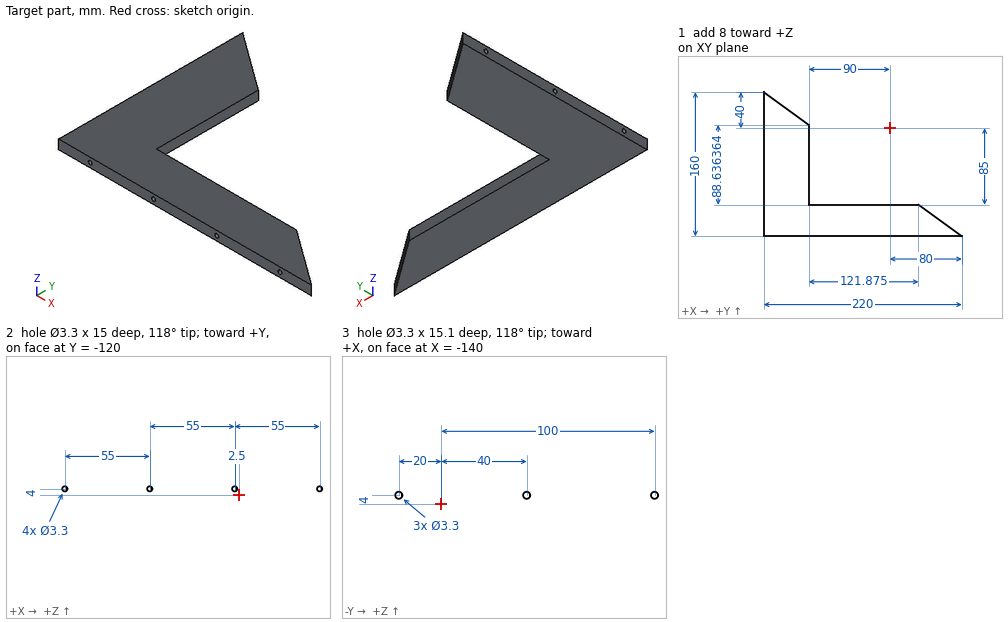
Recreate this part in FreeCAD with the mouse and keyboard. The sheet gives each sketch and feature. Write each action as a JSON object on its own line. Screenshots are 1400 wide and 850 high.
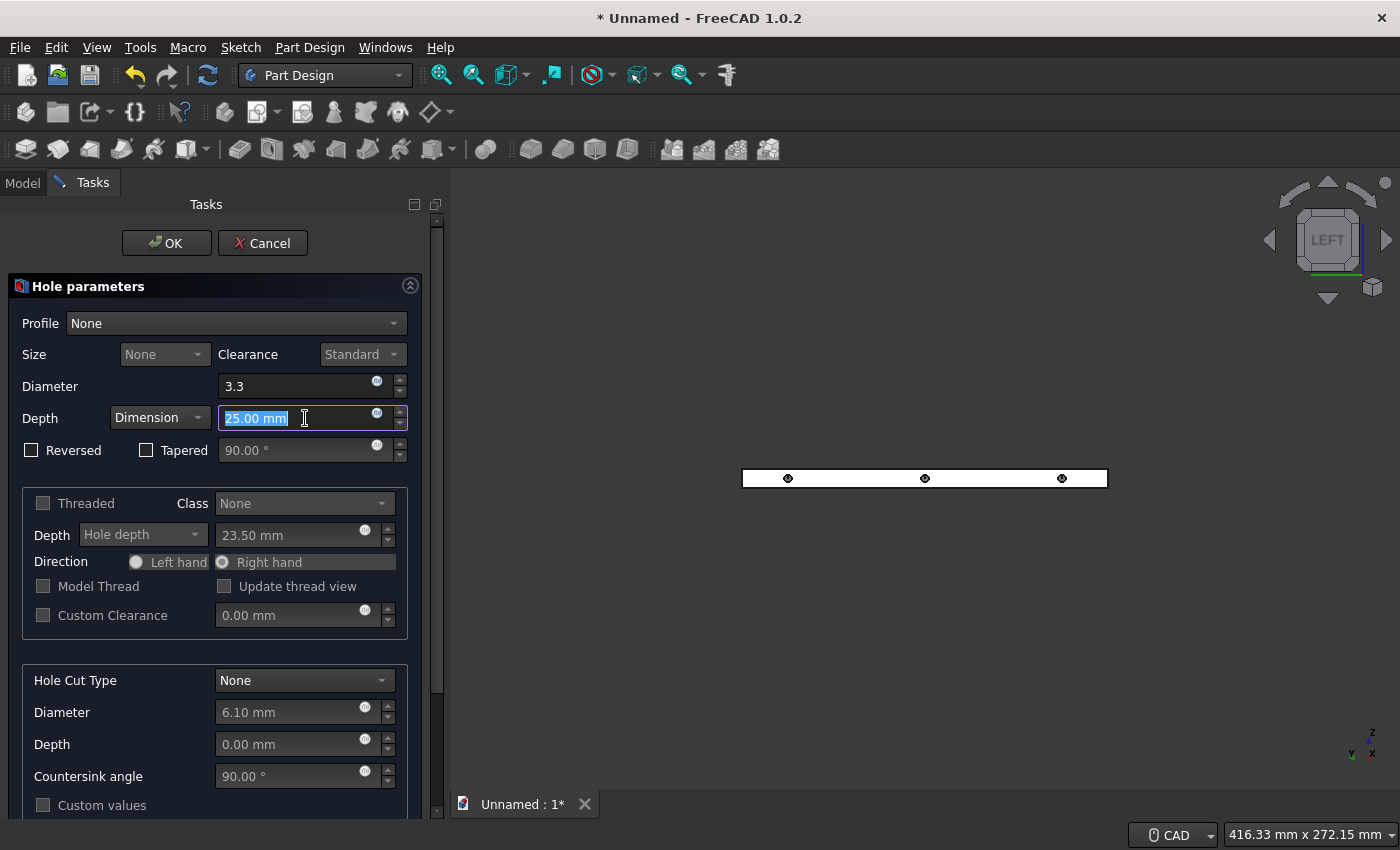
{"action": "type", "text": "15.1"}
{"action": "key", "text": "Tab"}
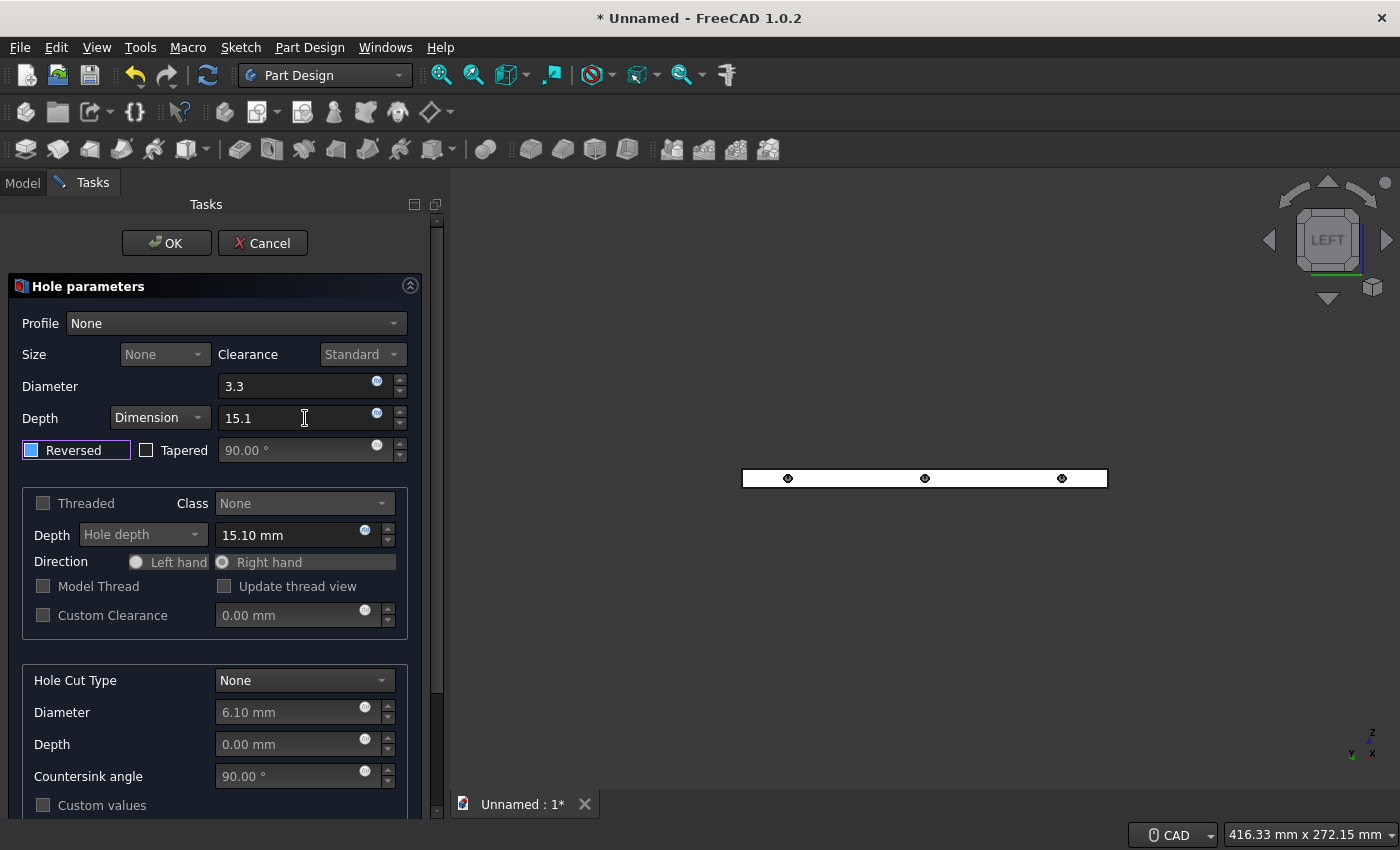
{"action": "left_click", "coordinate": [167, 243]}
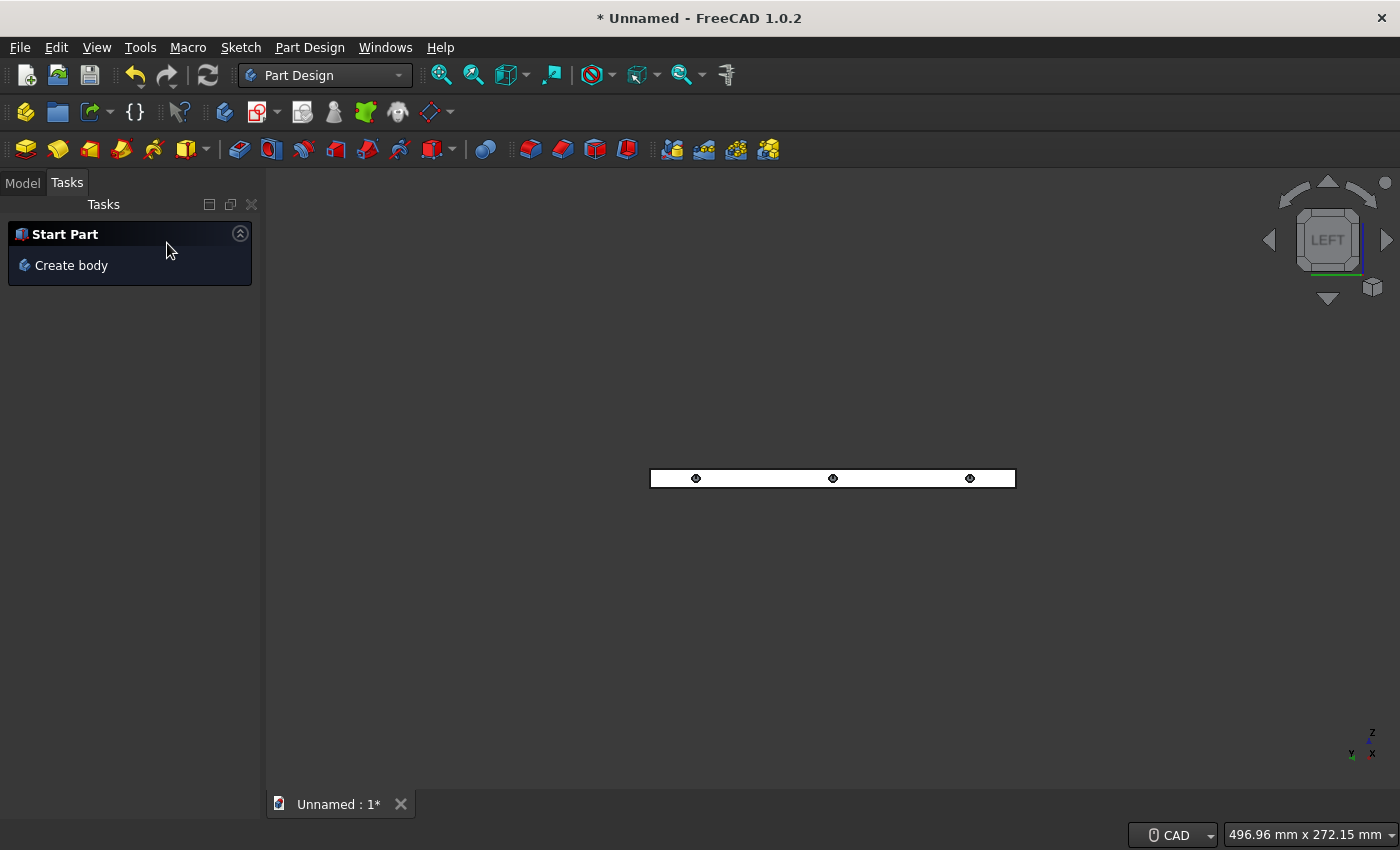
{"action": "key", "text": "0"}